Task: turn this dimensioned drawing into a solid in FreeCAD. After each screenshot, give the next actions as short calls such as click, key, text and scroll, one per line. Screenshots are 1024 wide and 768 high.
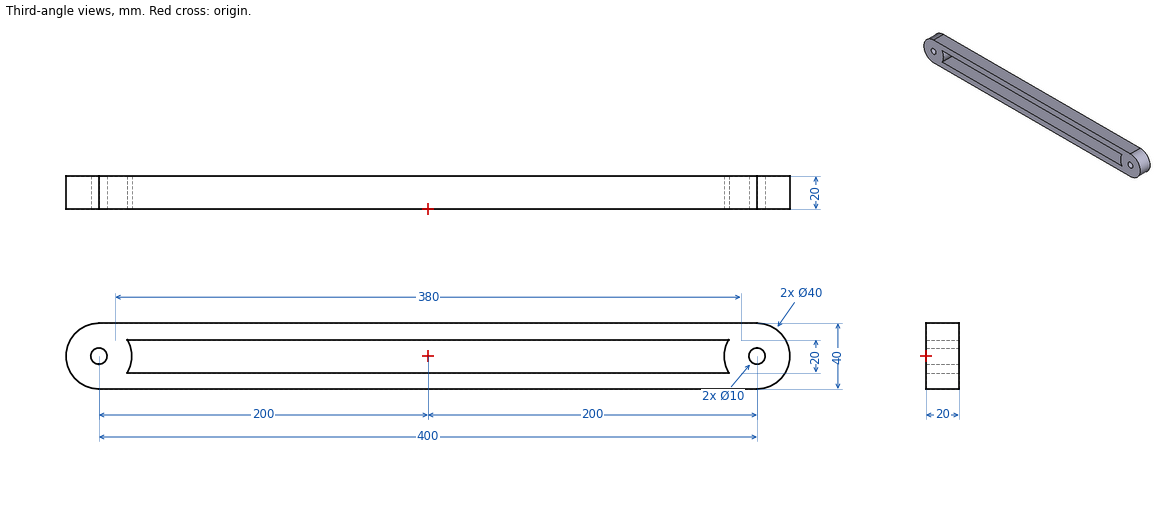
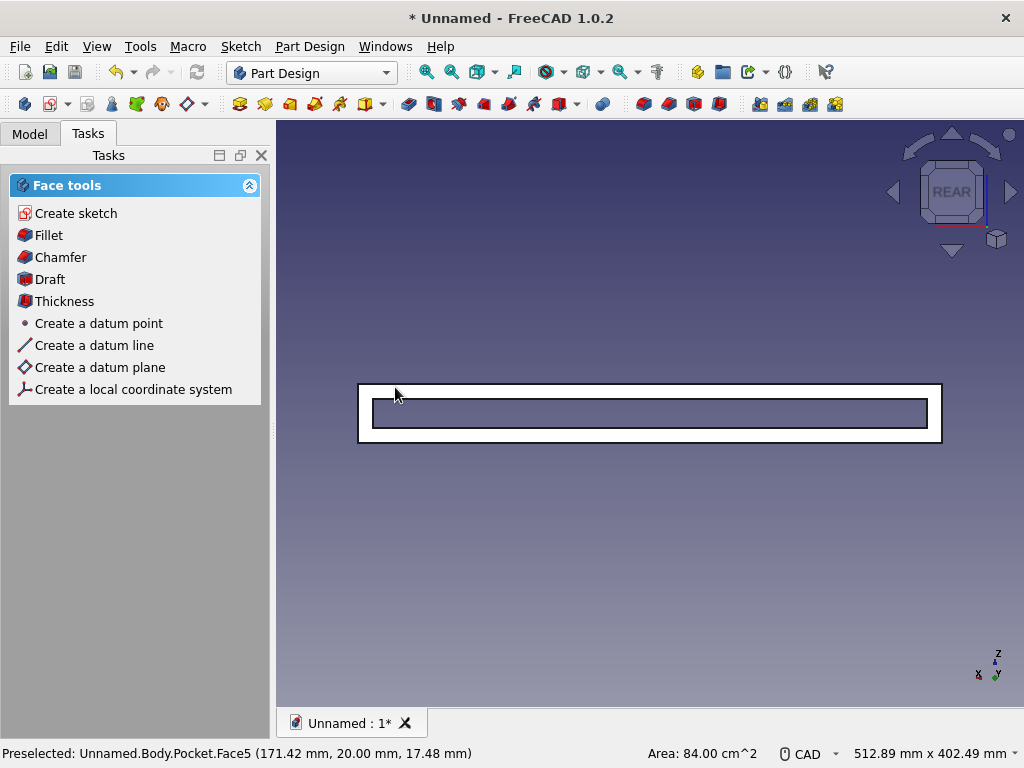
click(50, 104)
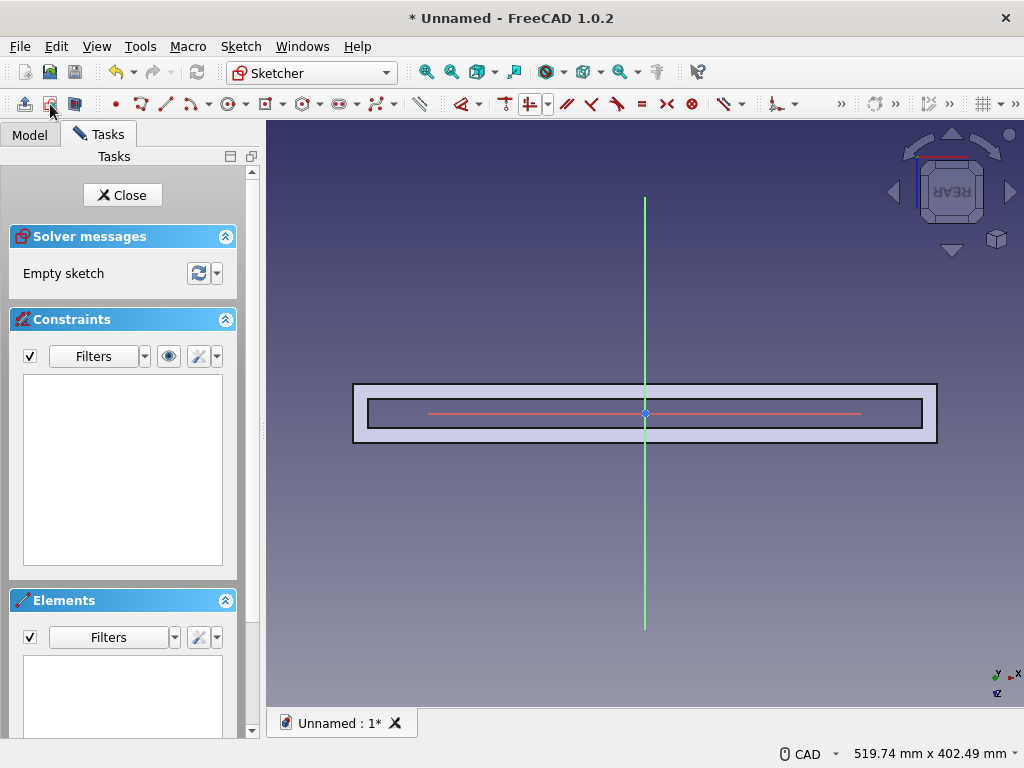
scroll(437, 414, down, 2)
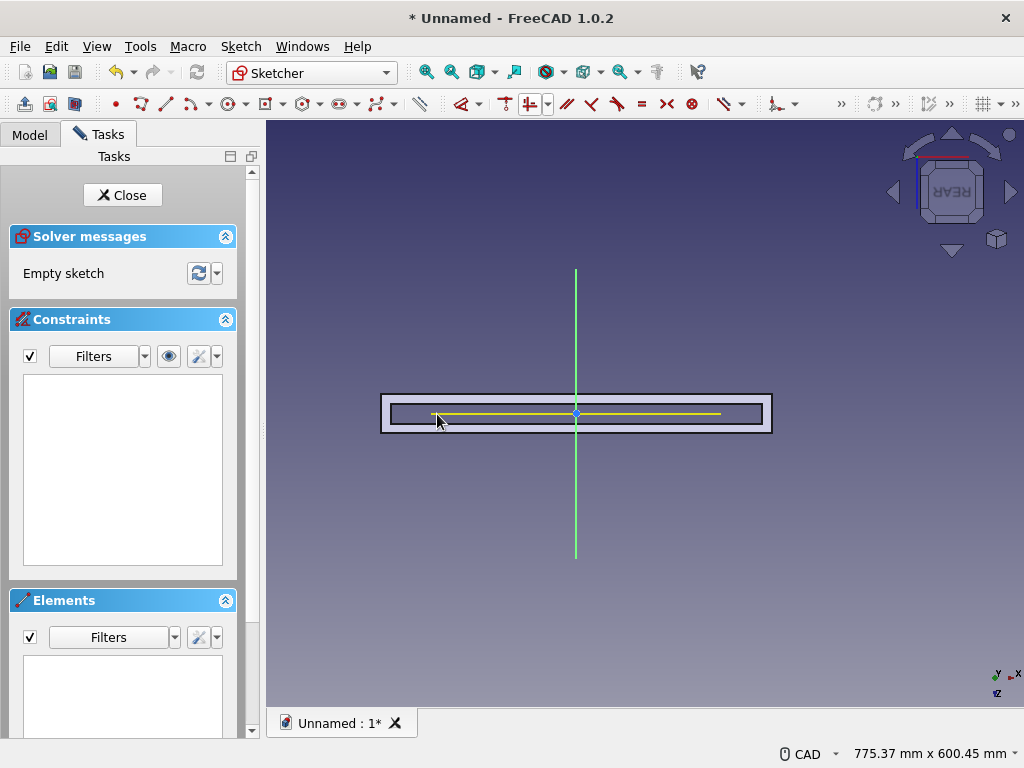
click(228, 104)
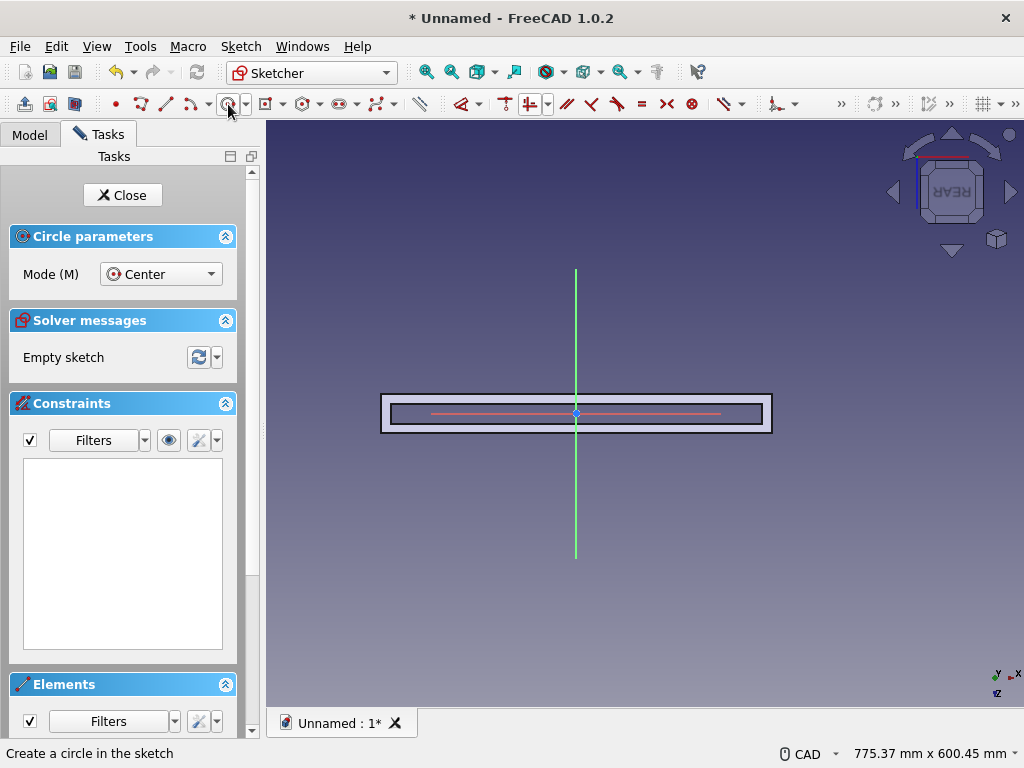
click(772, 414)
click(779, 395)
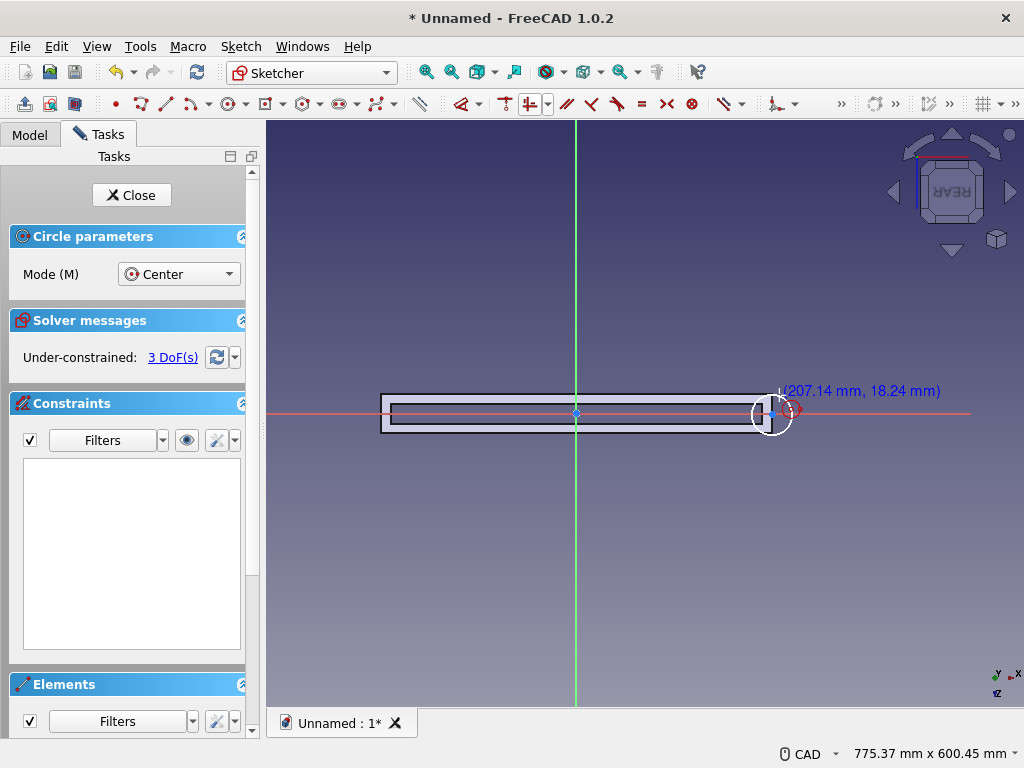
click(381, 414)
click(388, 395)
key(Escape)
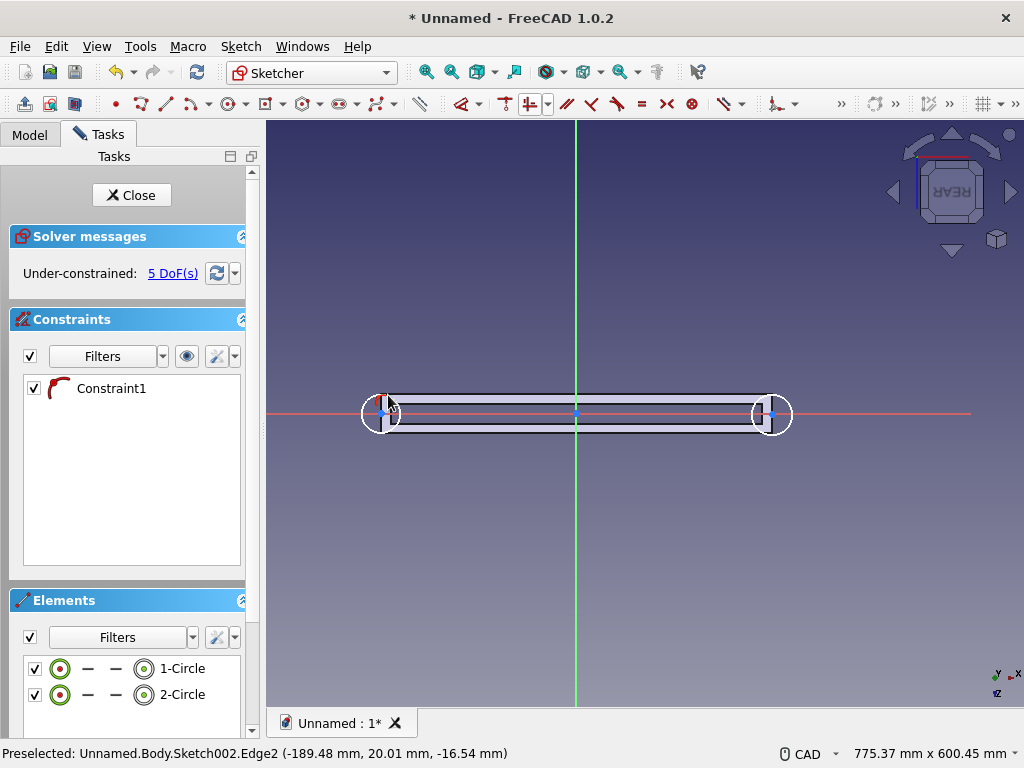
click(786, 401)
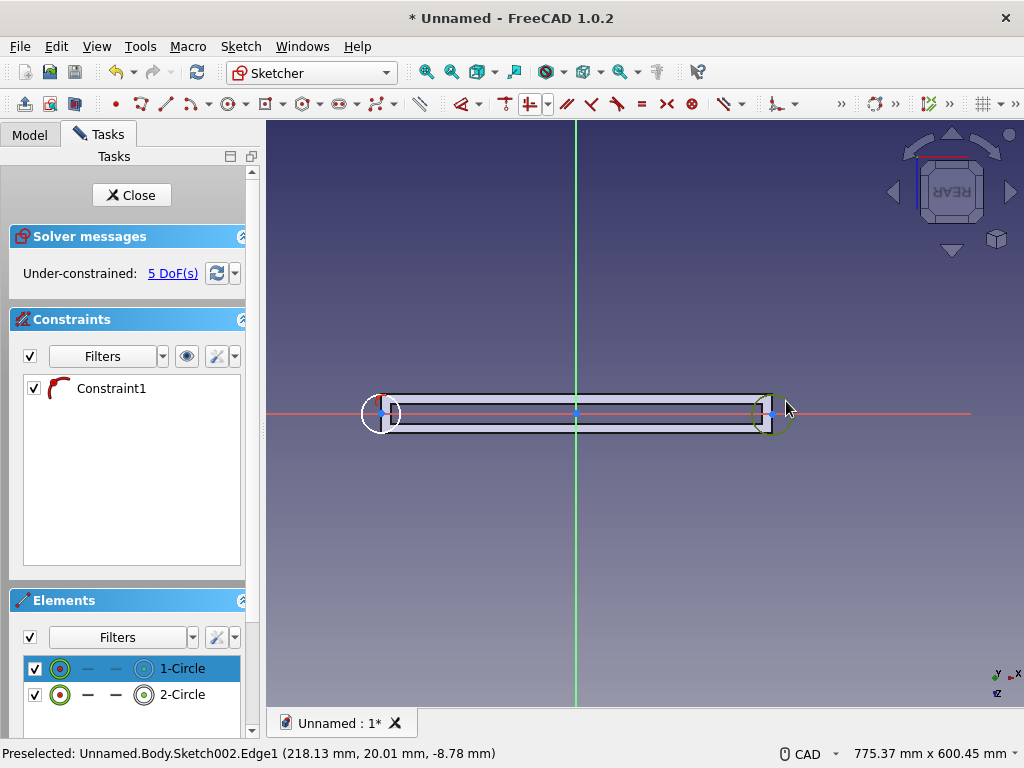
click(395, 400)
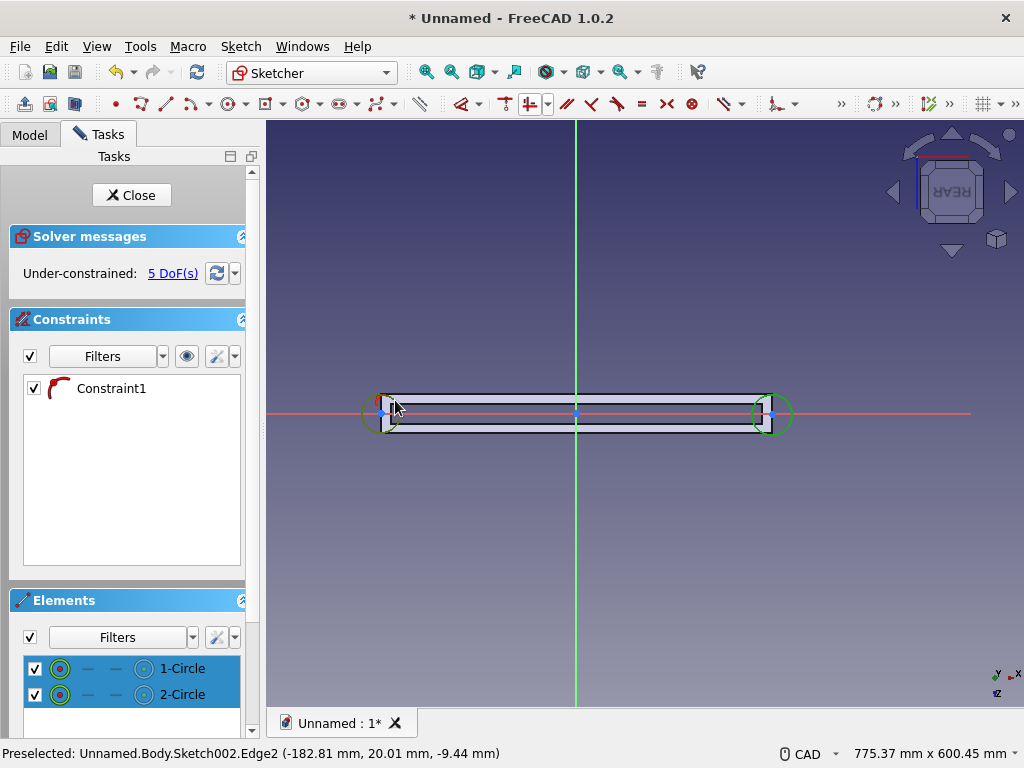
click(642, 104)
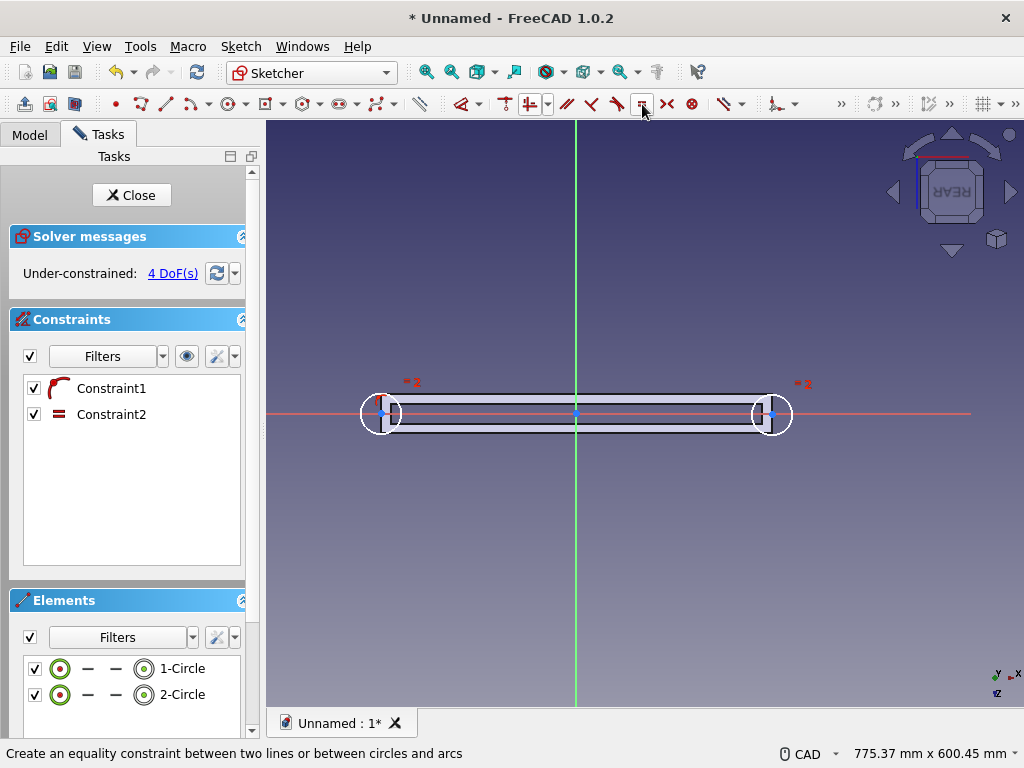
click(772, 415)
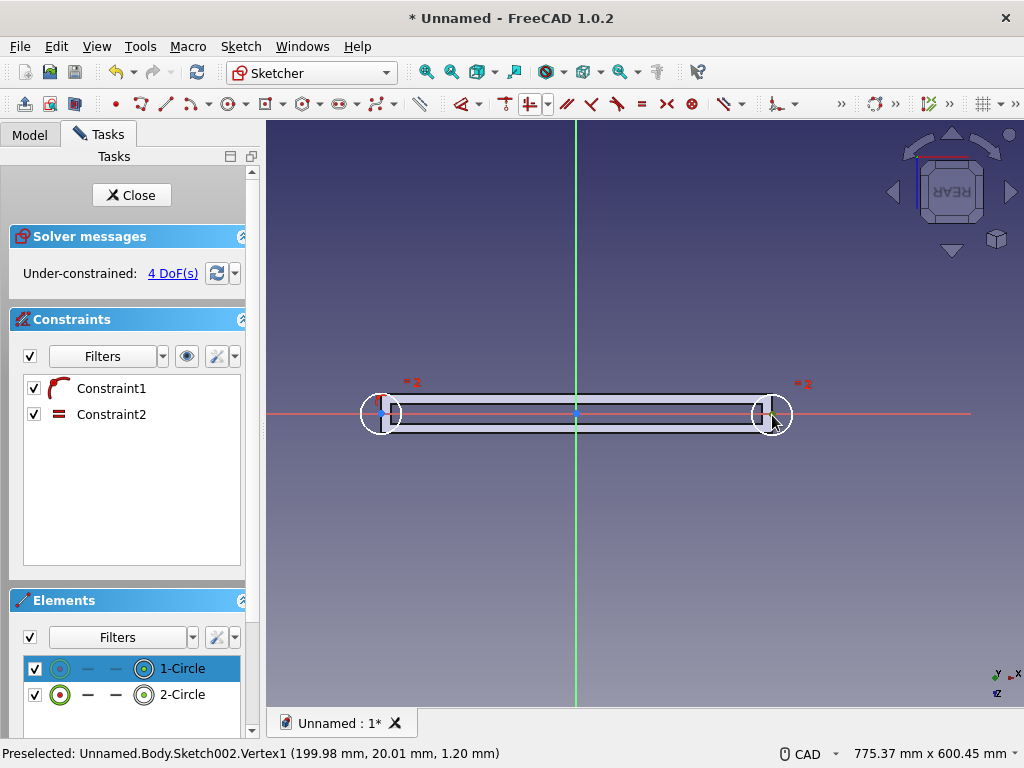
click(455, 414)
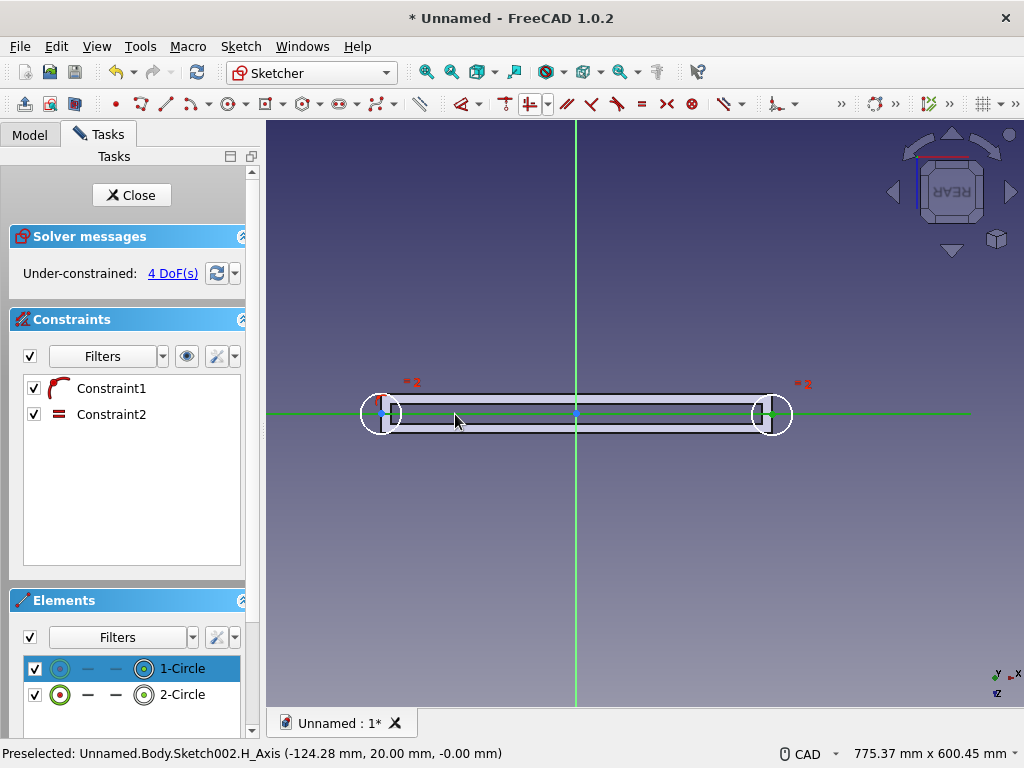
click(505, 104)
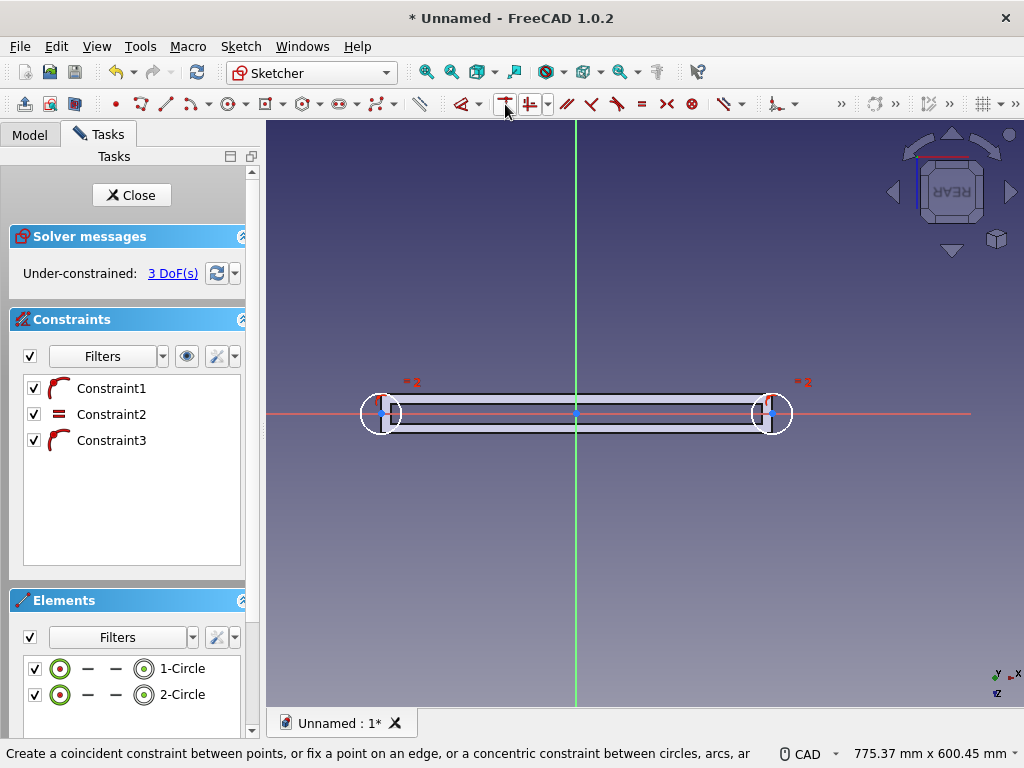
click(460, 104)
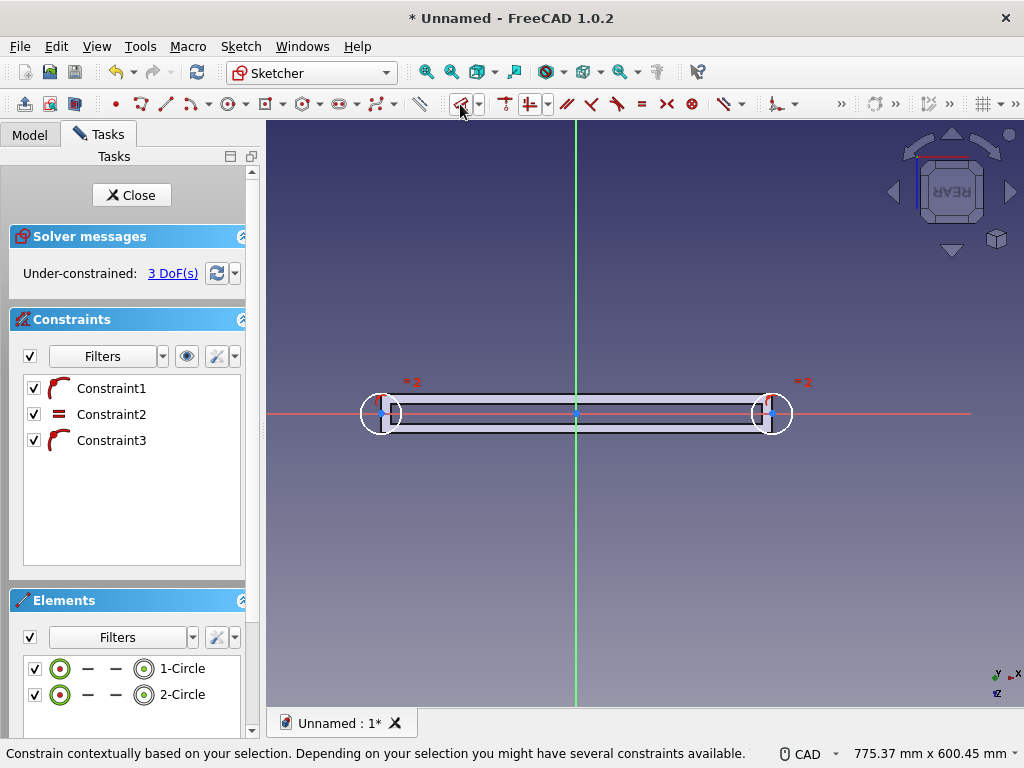
click(786, 399)
click(808, 376)